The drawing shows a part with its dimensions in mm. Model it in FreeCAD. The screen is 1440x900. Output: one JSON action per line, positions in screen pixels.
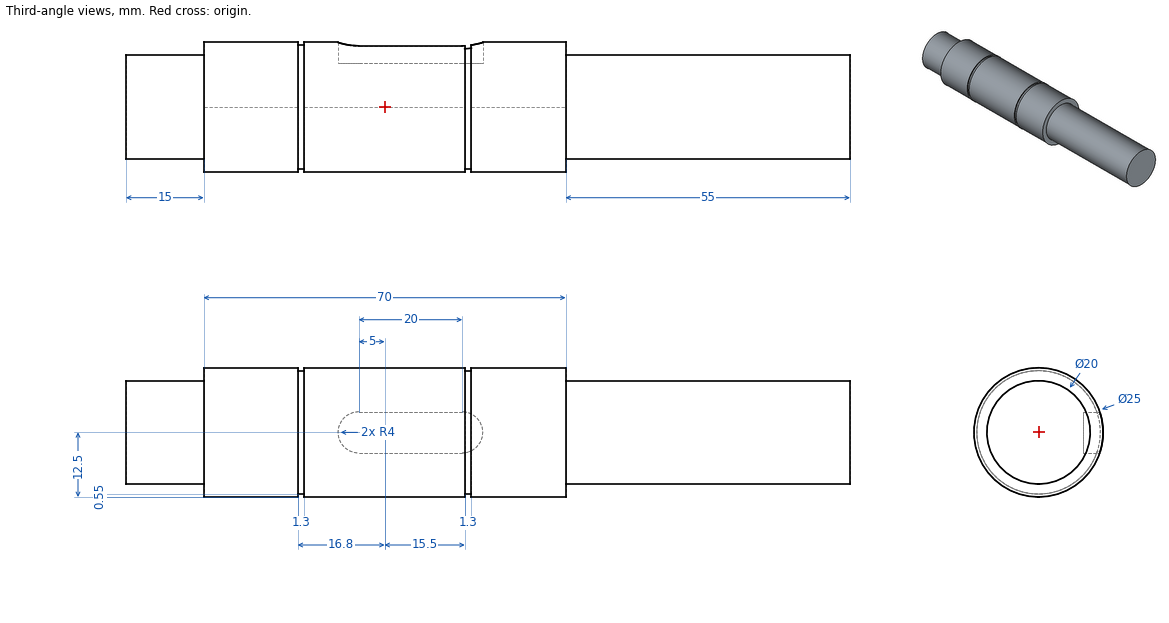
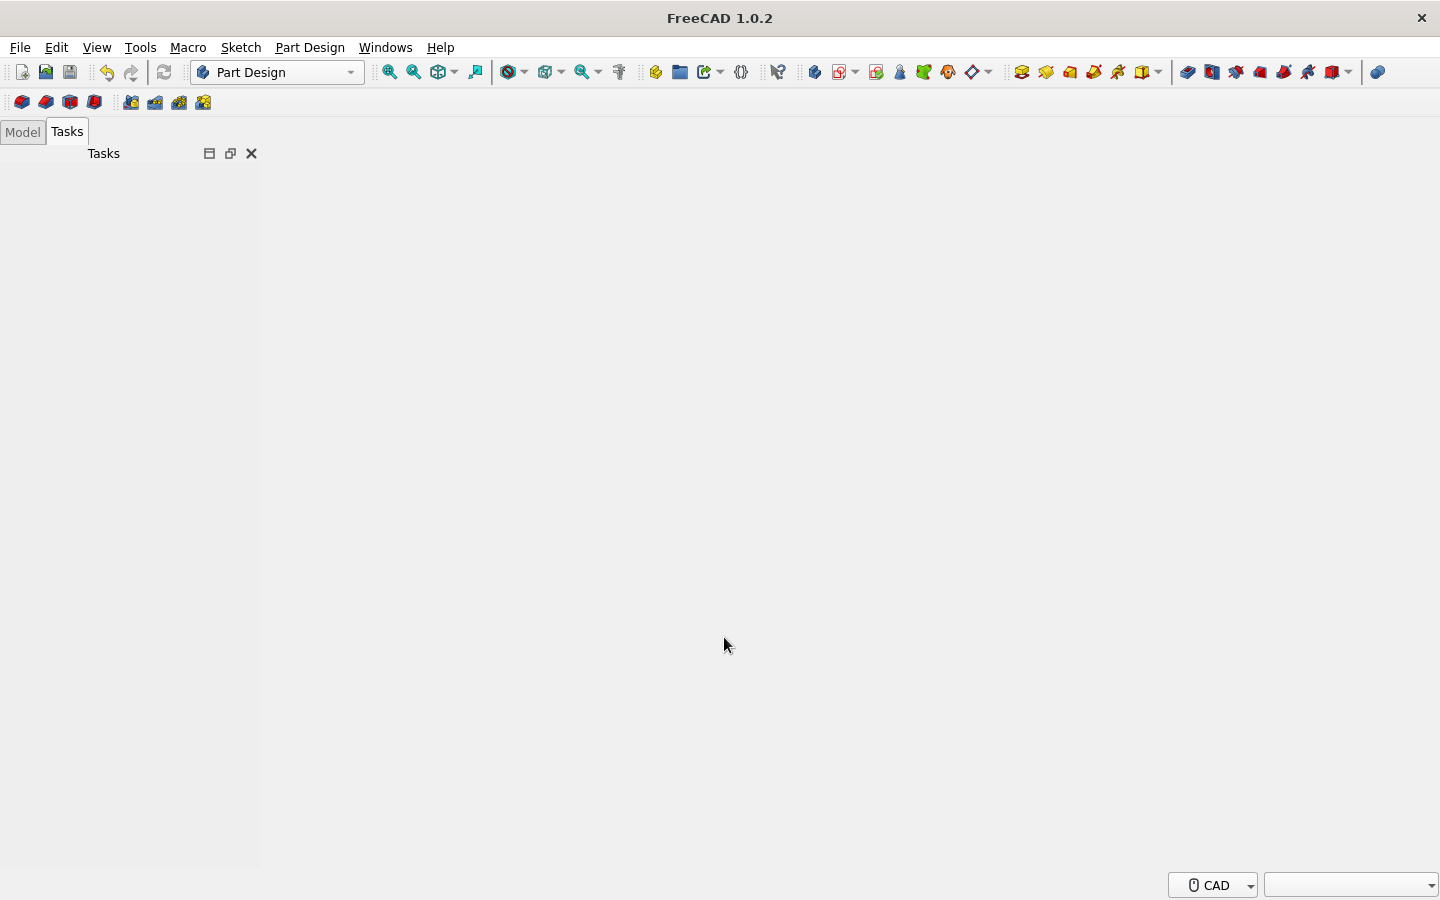
{"action": "key", "text": "ctrl+n"}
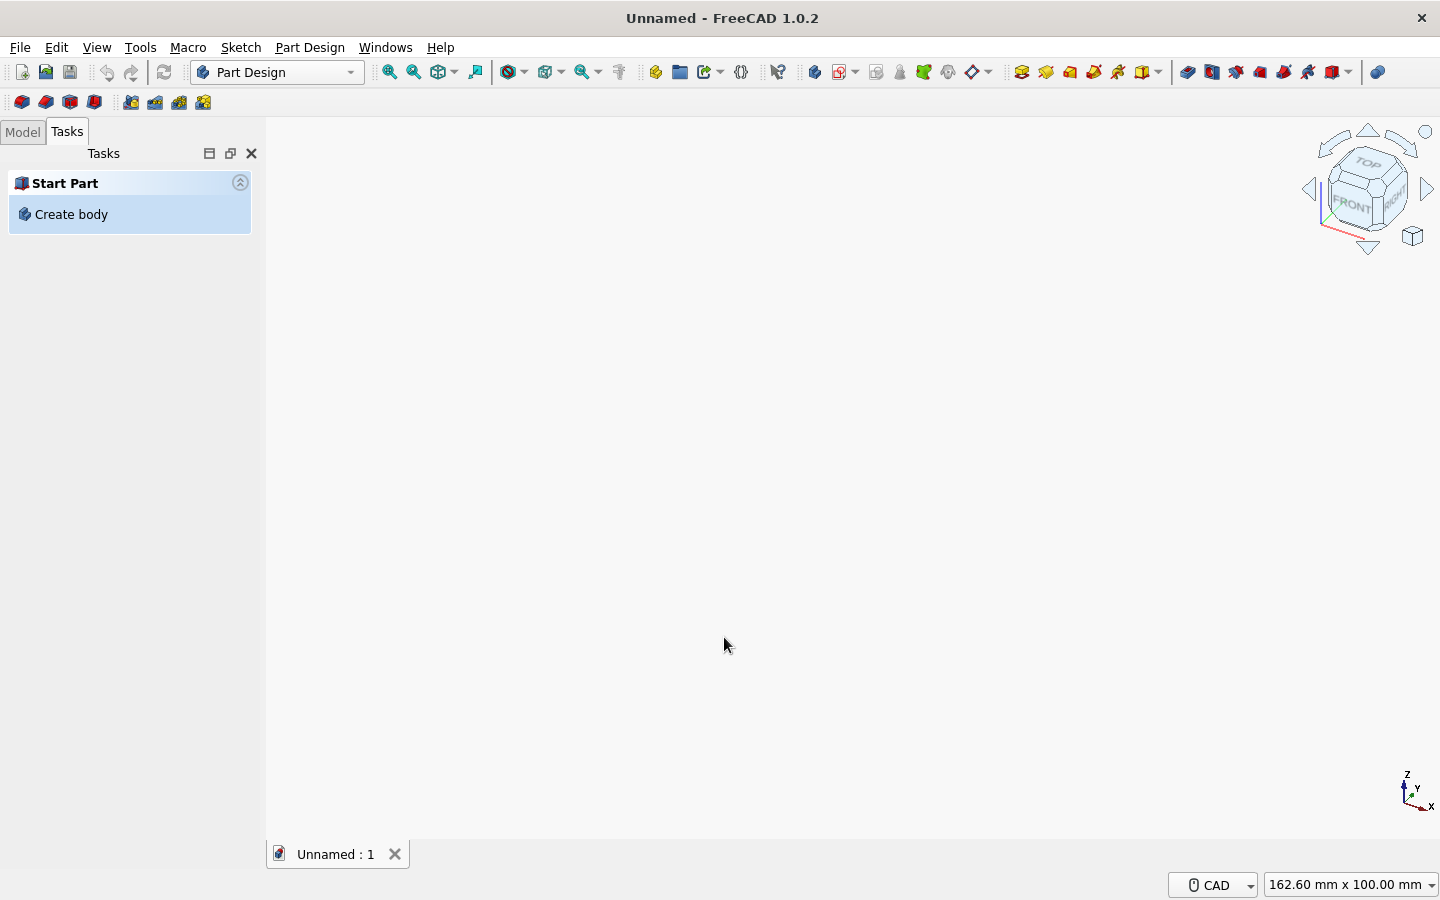
{"action": "left_click", "coordinate": [840, 72]}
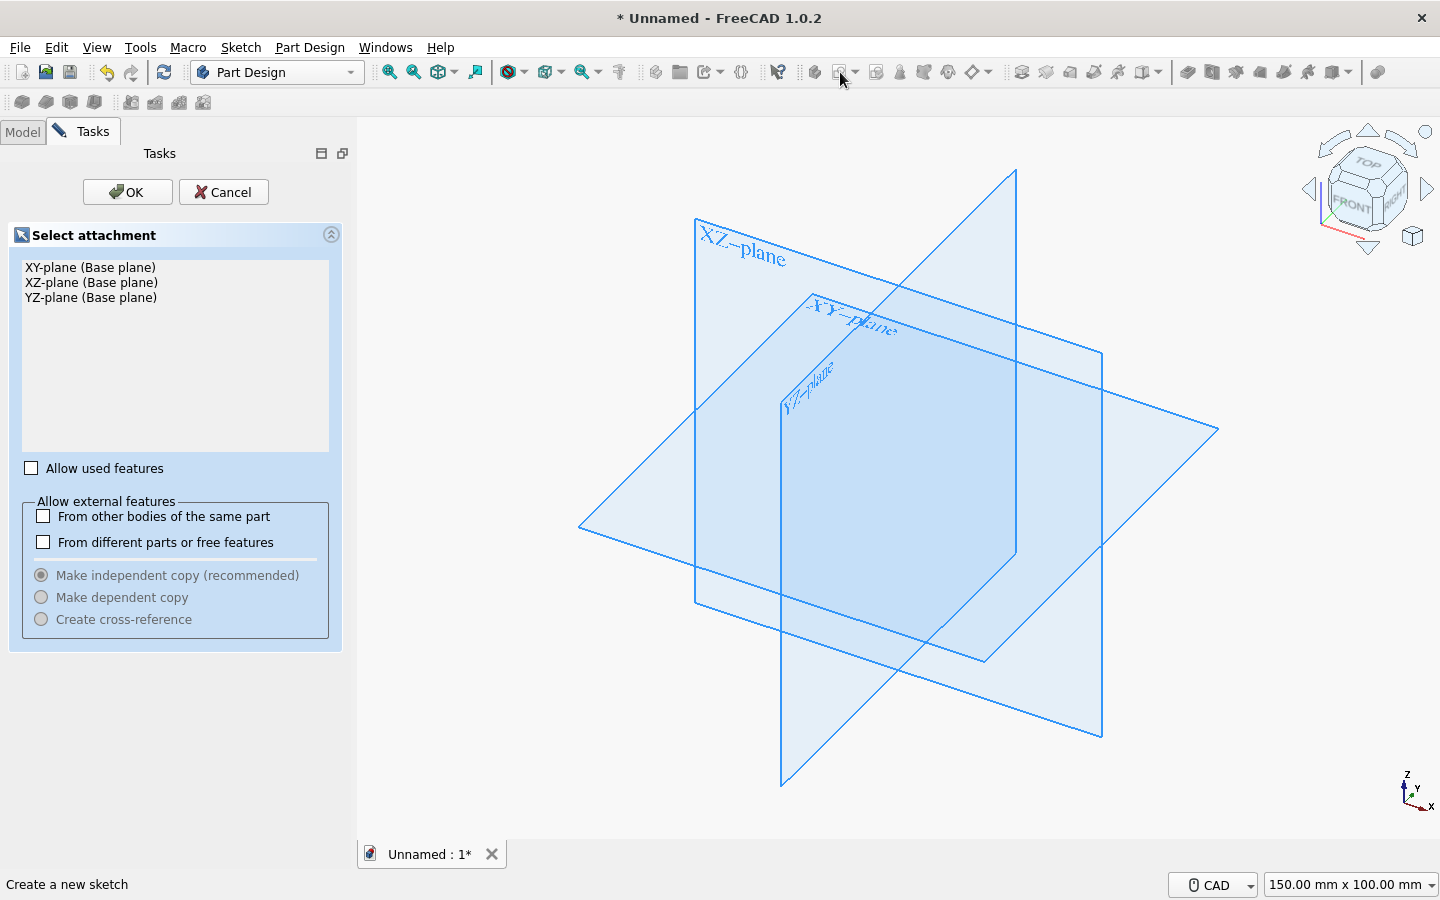
{"action": "left_click", "coordinate": [82, 298]}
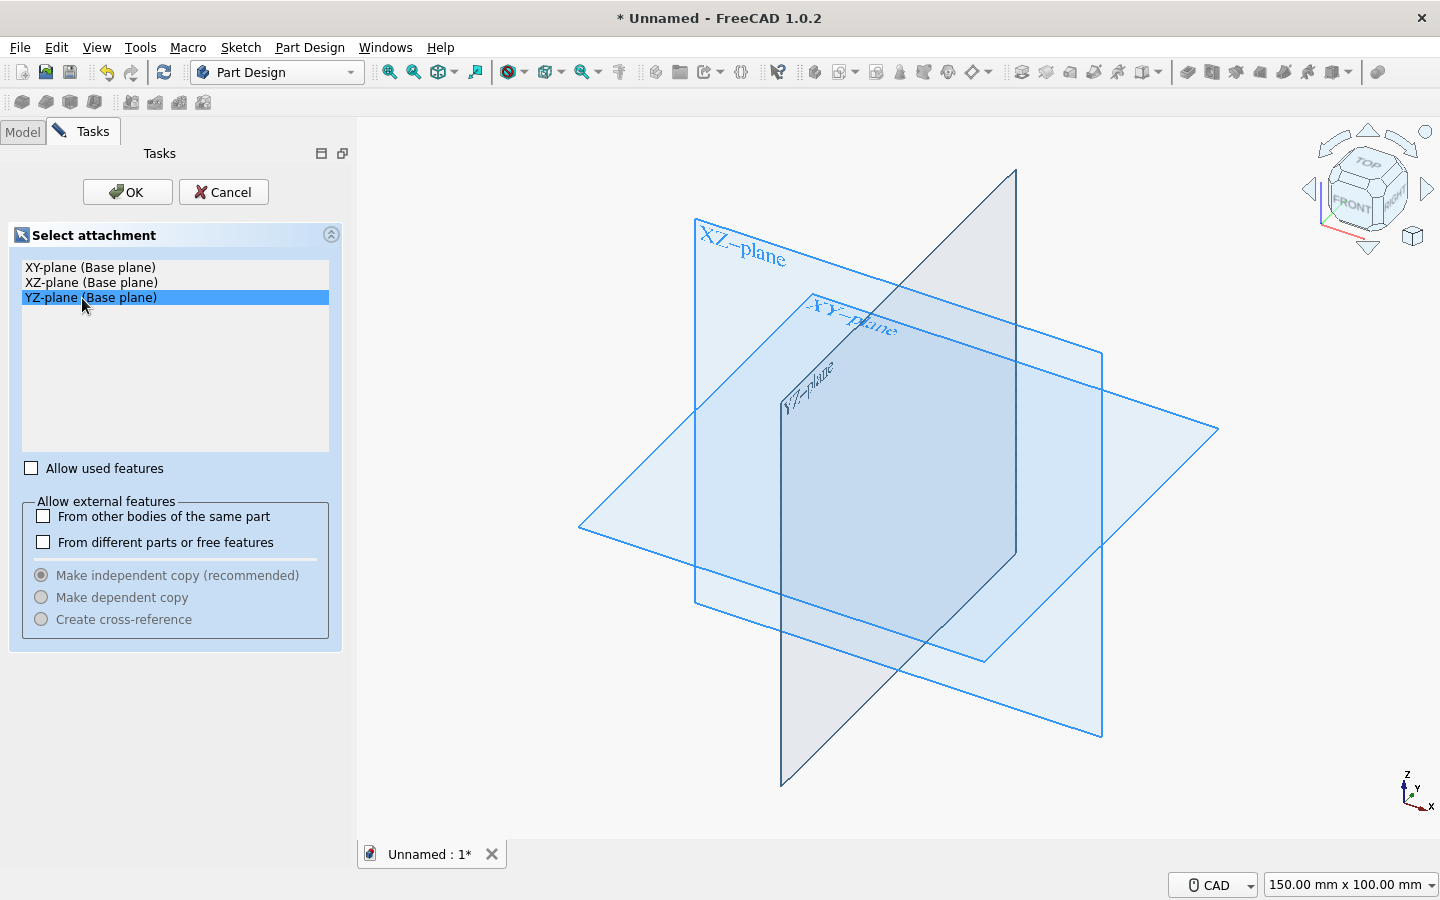
{"action": "left_click", "coordinate": [128, 192]}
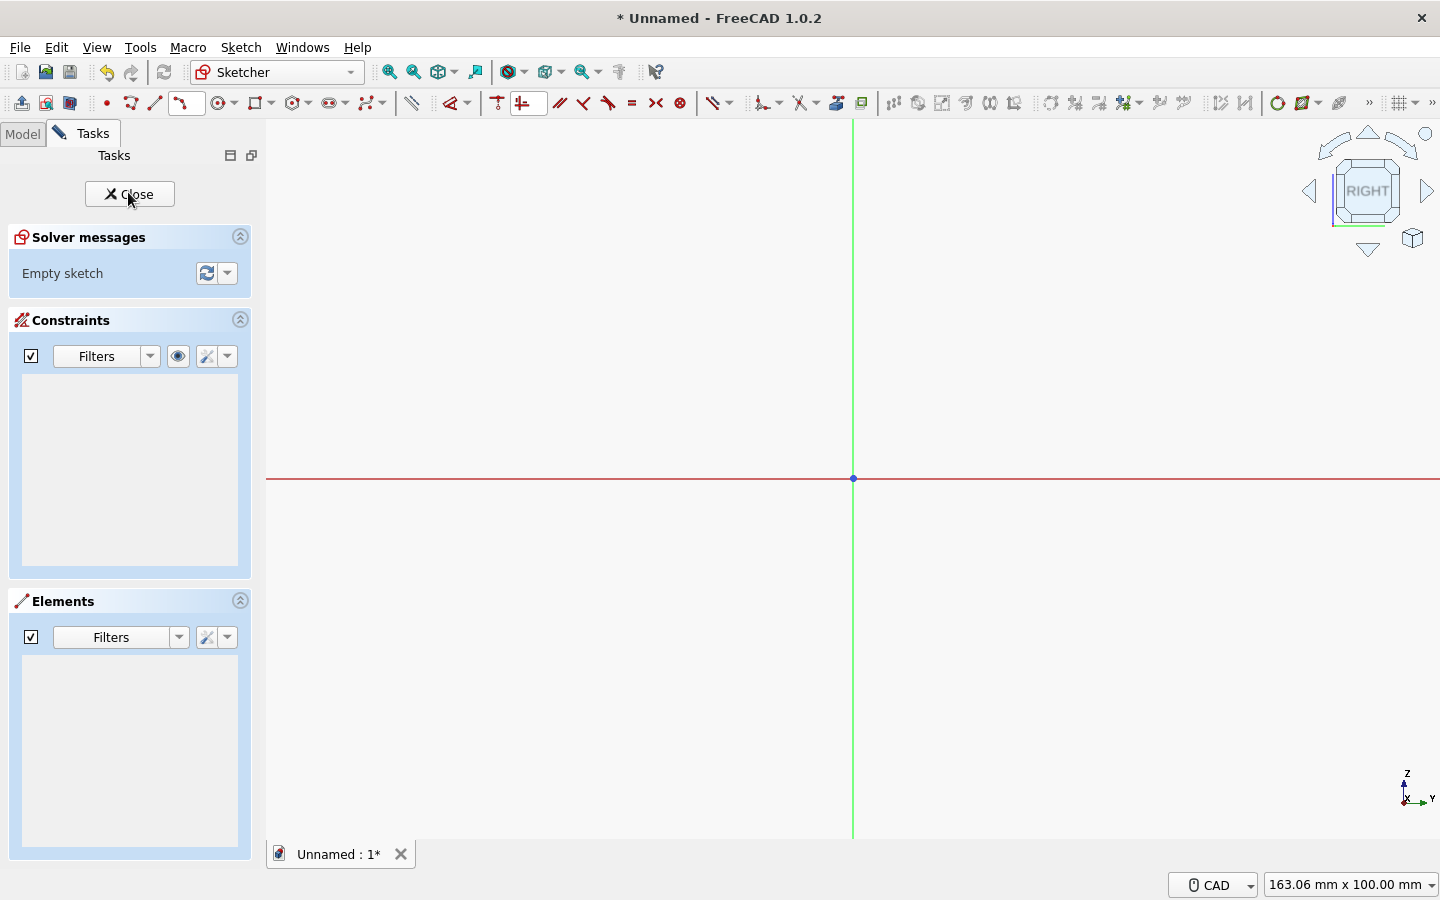
{"action": "scroll", "coordinate": [893, 479], "scroll_direction": "up", "scroll_amount": 5}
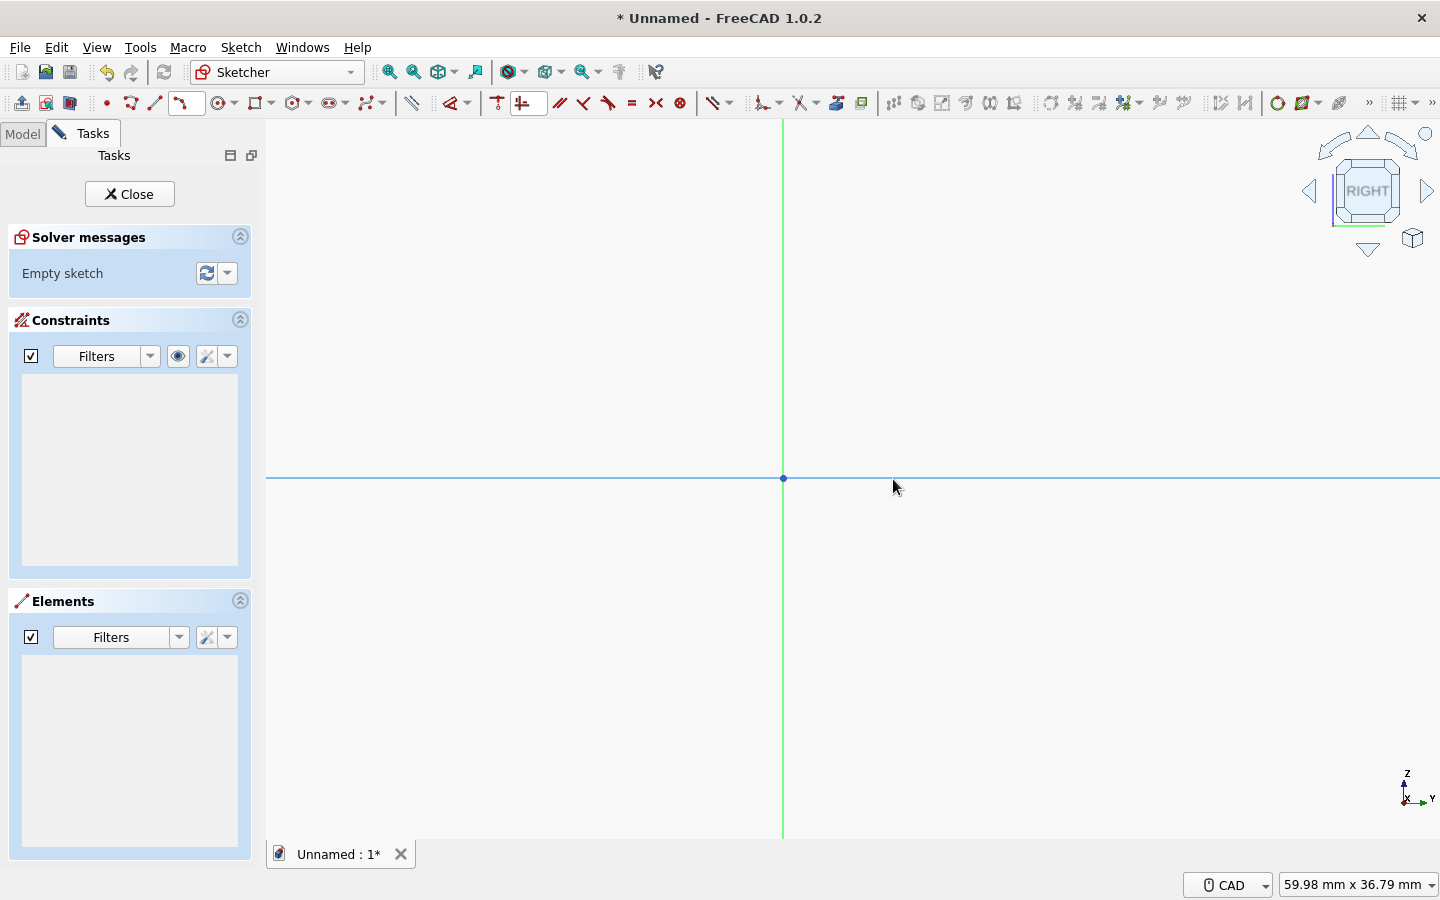
{"action": "left_click", "coordinate": [218, 104]}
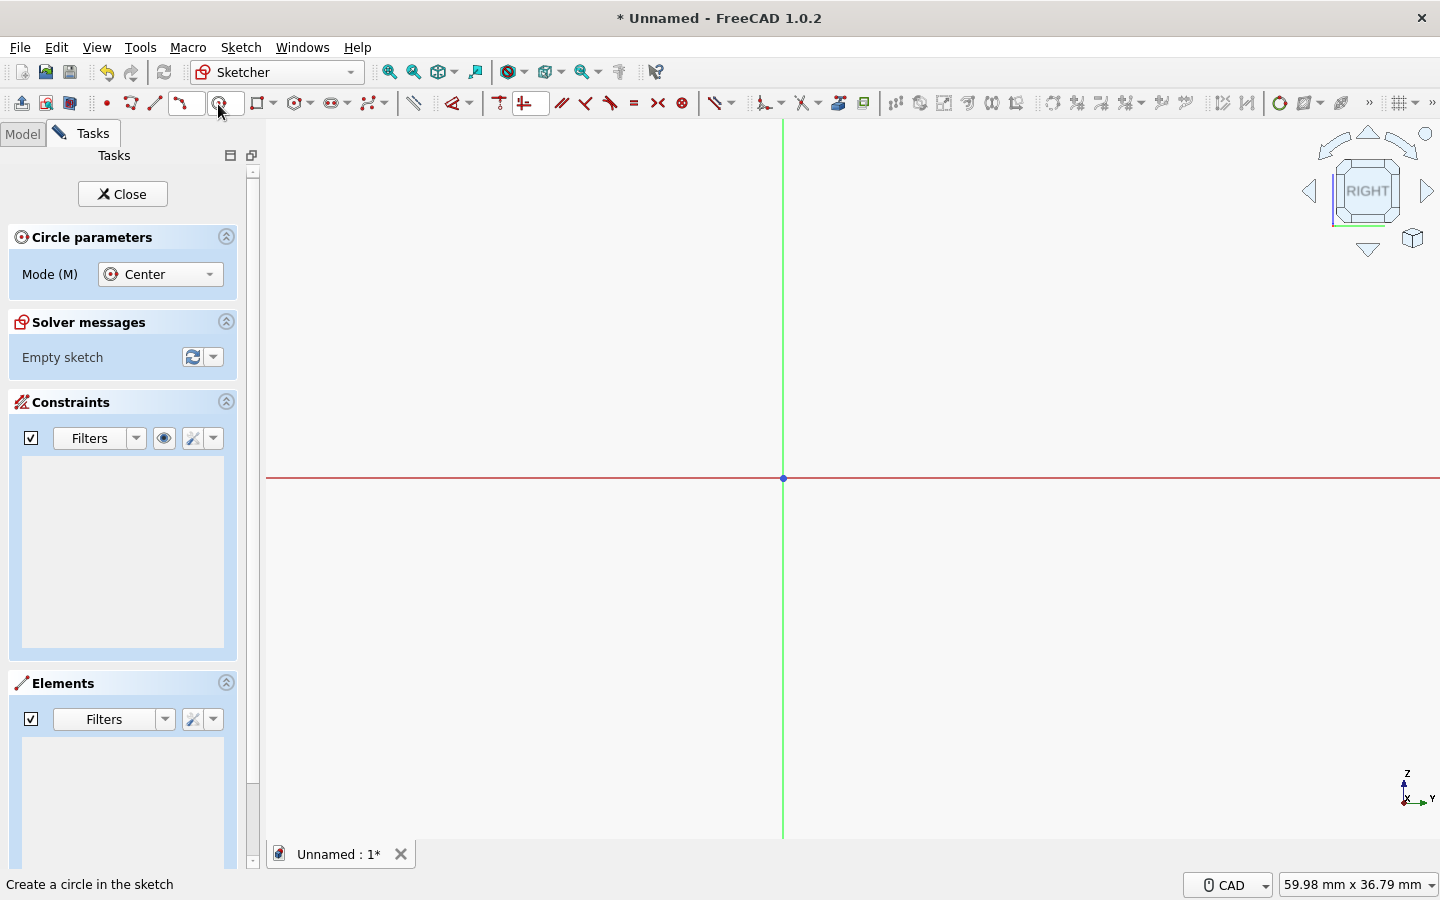
{"action": "left_click", "coordinate": [783, 478]}
{"action": "left_click", "coordinate": [956, 305]}
{"action": "key", "text": "Escape"}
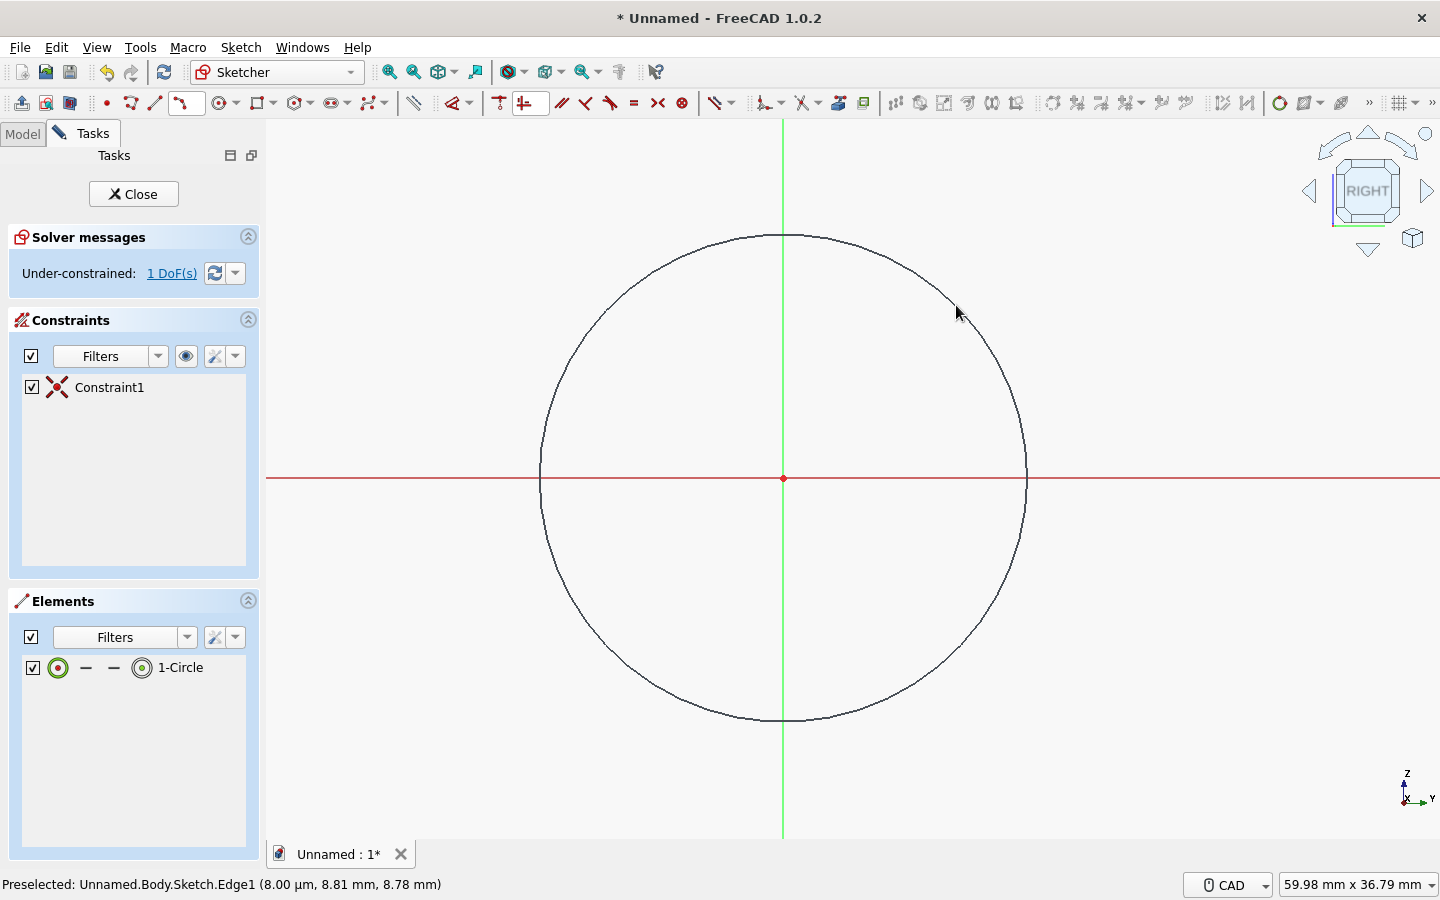
{"action": "left_click", "coordinate": [955, 305]}